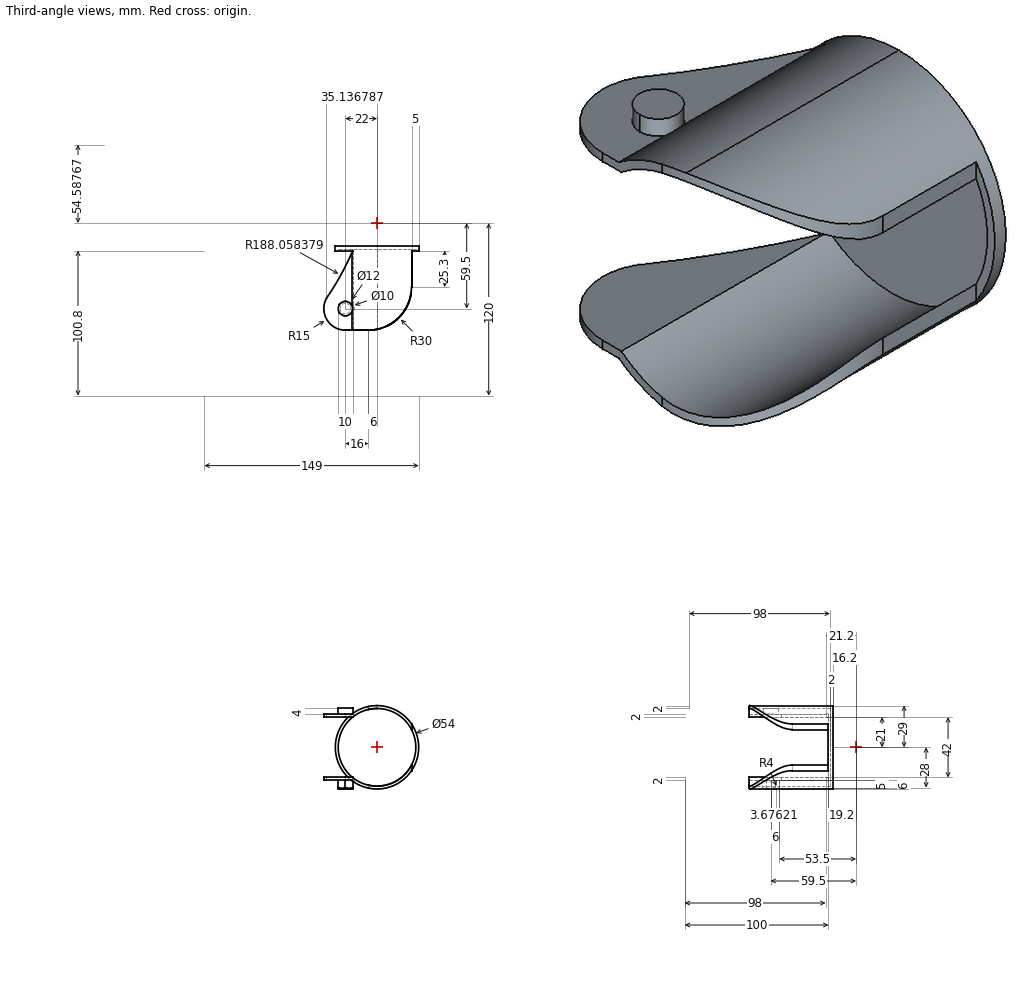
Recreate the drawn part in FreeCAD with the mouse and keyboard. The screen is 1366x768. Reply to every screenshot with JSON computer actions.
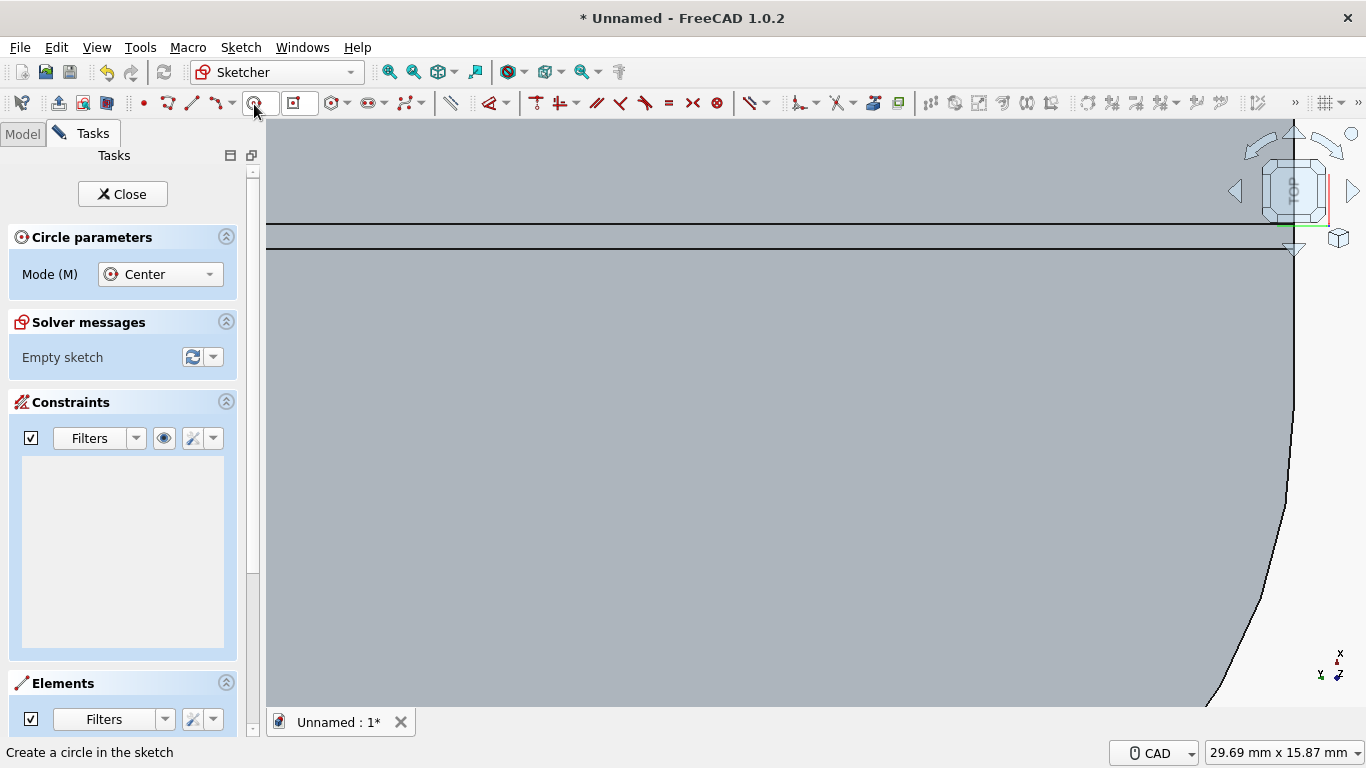
{"action": "left_click", "coordinate": [738, 410]}
{"action": "left_click", "coordinate": [869, 279]}
{"action": "key", "text": "Escape"}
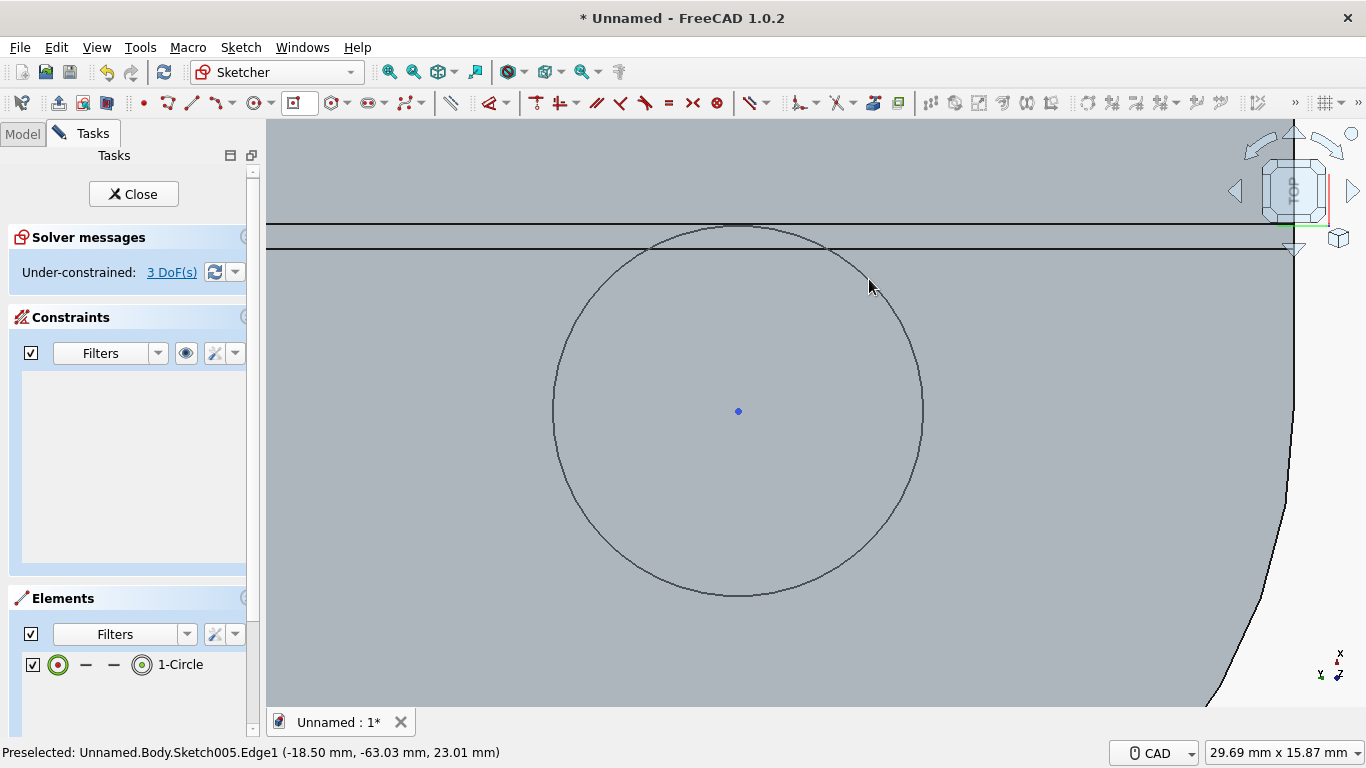
{"action": "left_click", "coordinate": [490, 104]}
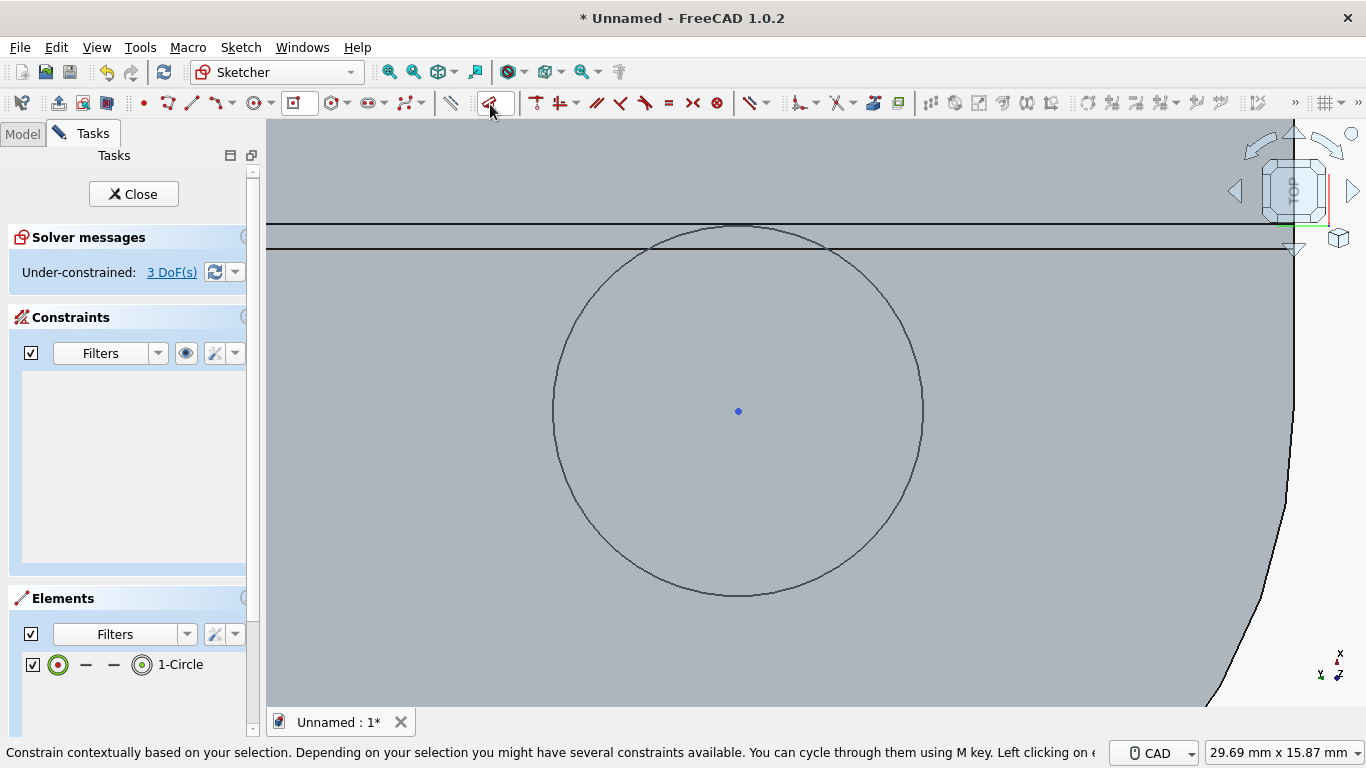
{"action": "left_click", "coordinate": [869, 280]}
{"action": "left_click", "coordinate": [892, 257]}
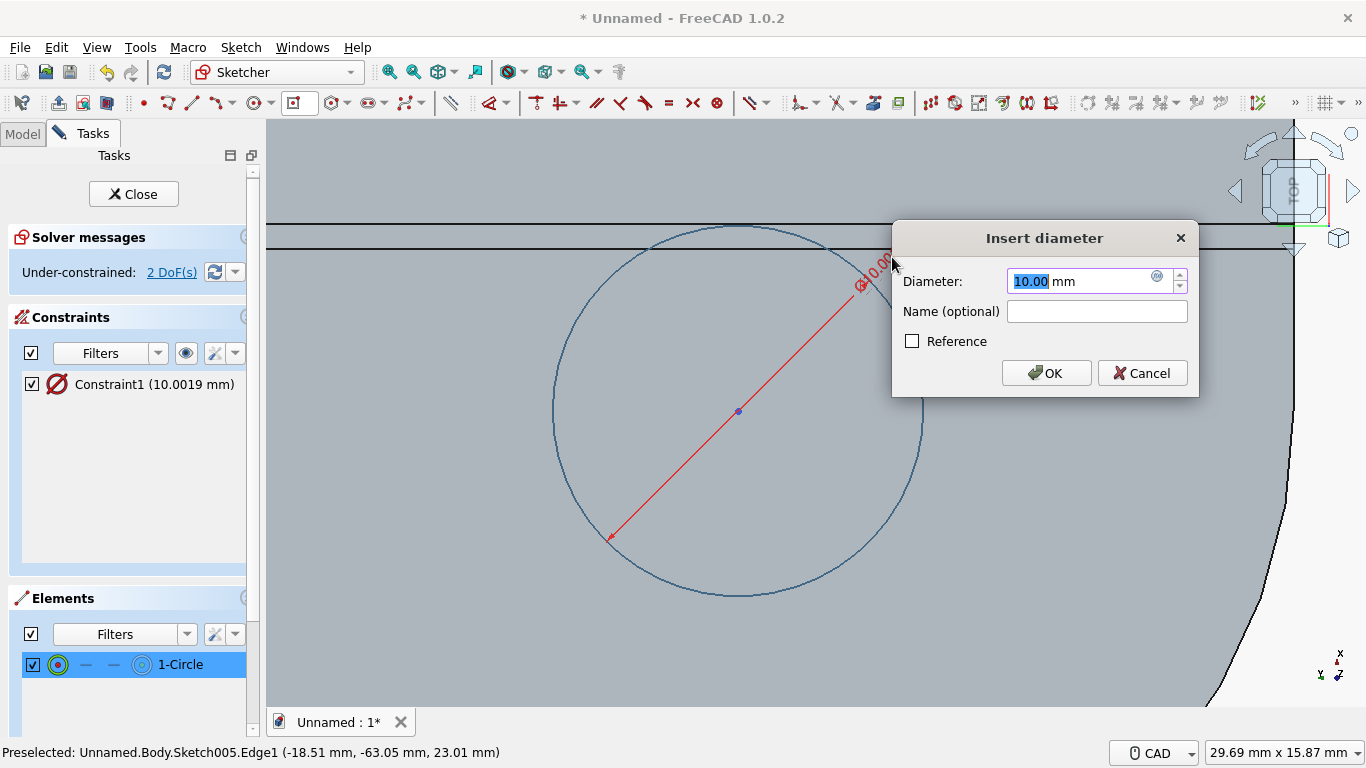
{"action": "type", "text": "10"}
{"action": "key", "text": "Return"}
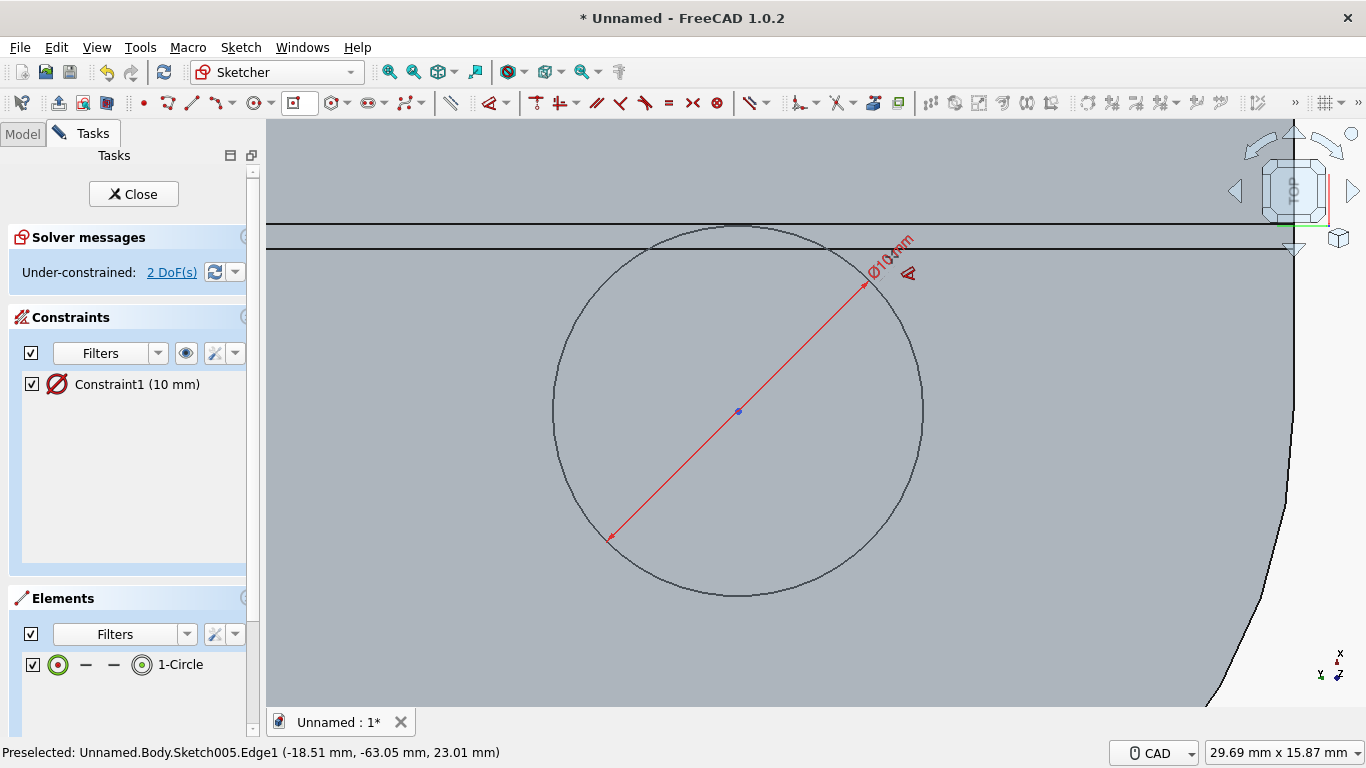
{"action": "left_click", "coordinate": [738, 411]}
{"action": "left_click", "coordinate": [772, 279]}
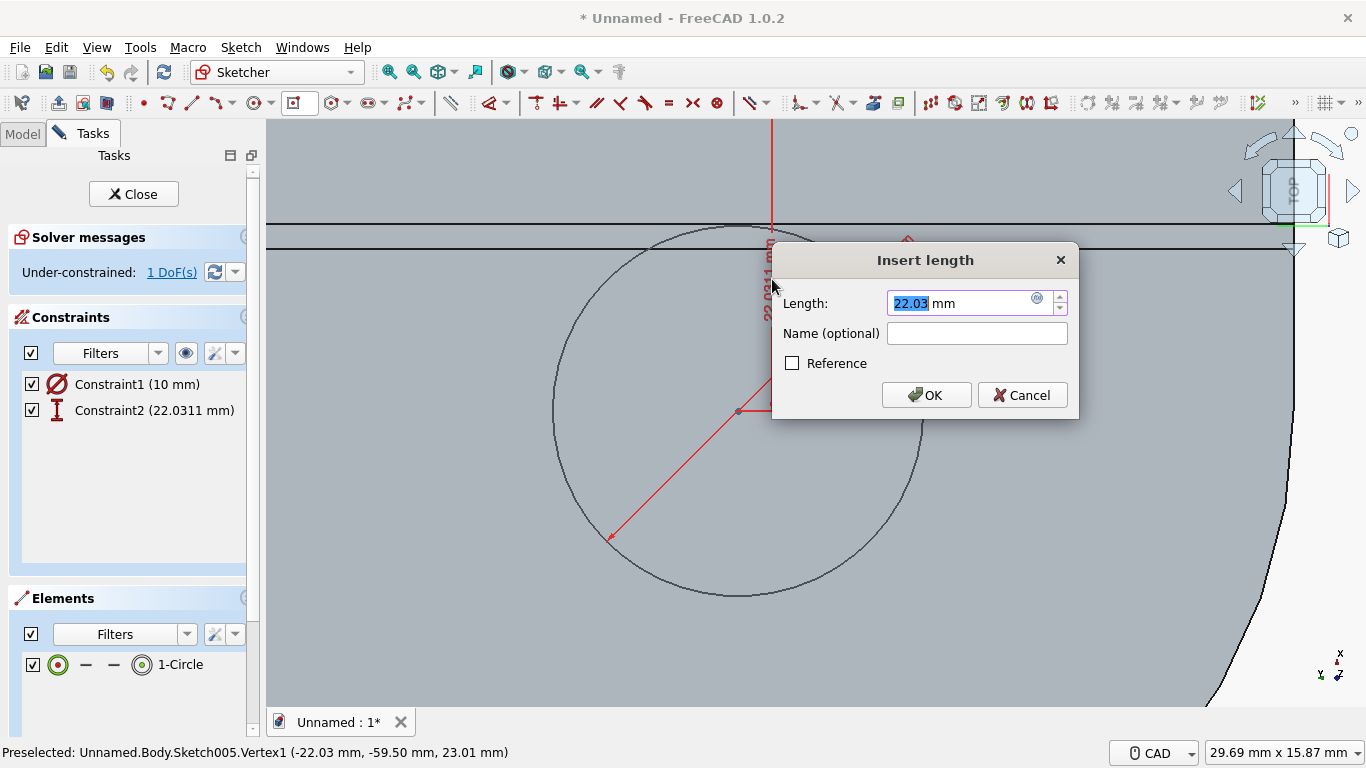
{"action": "type", "text": "22"}
{"action": "key", "text": "Return"}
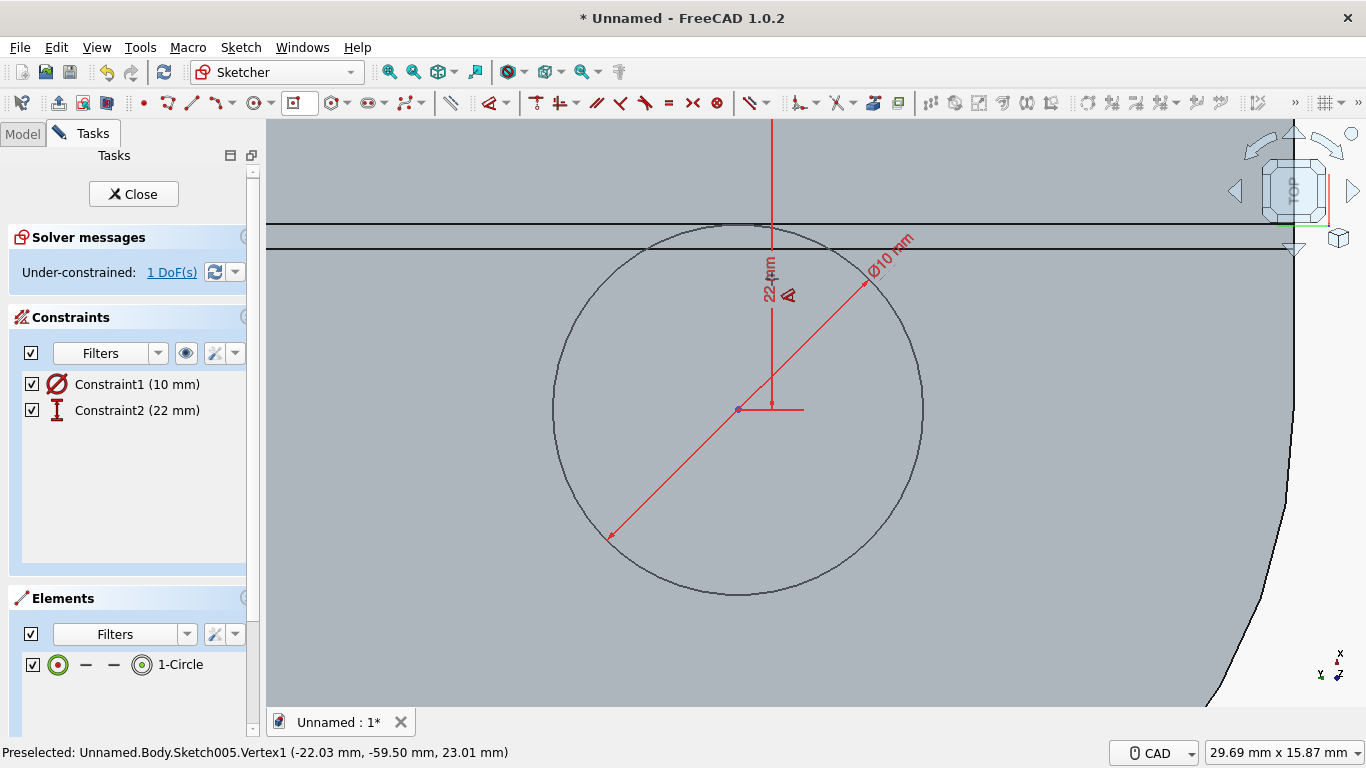
{"action": "left_click", "coordinate": [738, 410]}
{"action": "left_click", "coordinate": [516, 444]}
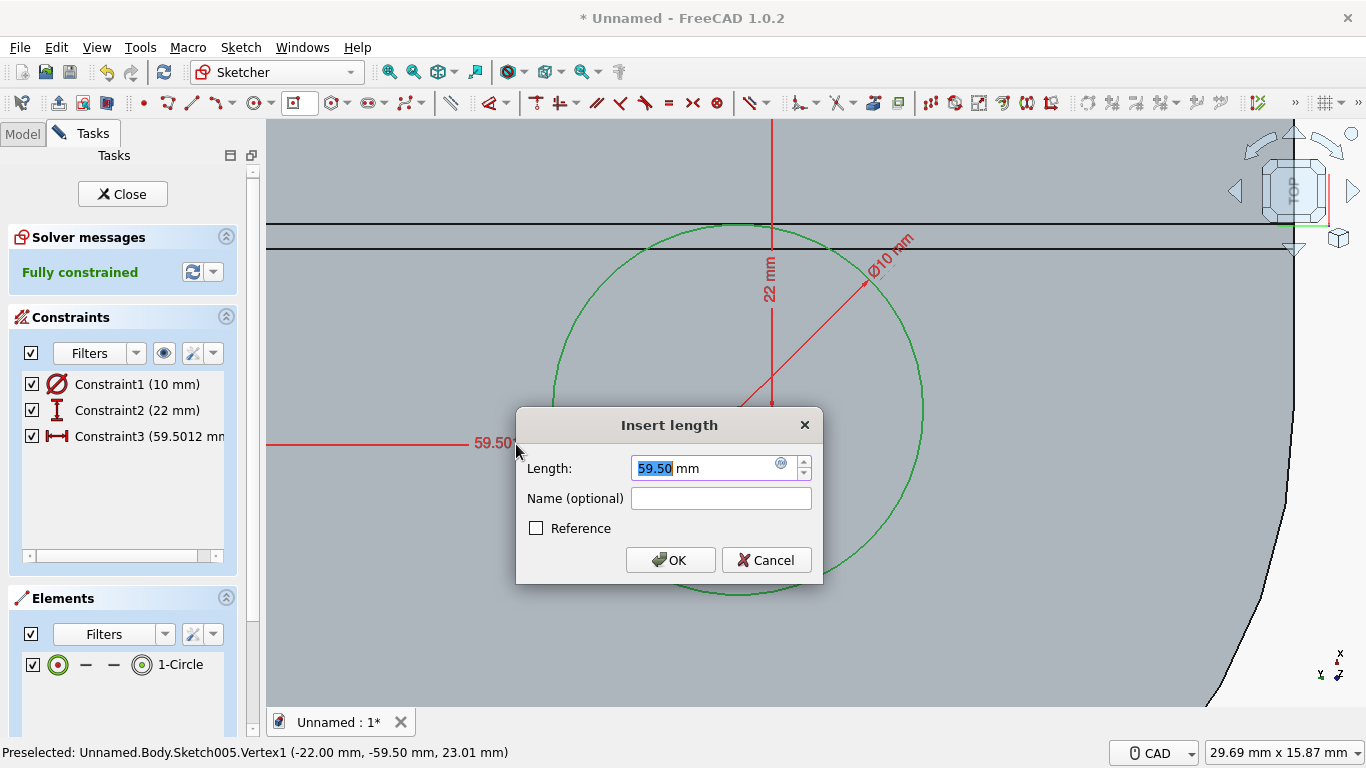
{"action": "type", "text": "59.5"}
{"action": "key", "text": "Return"}
{"action": "key", "text": "Escape"}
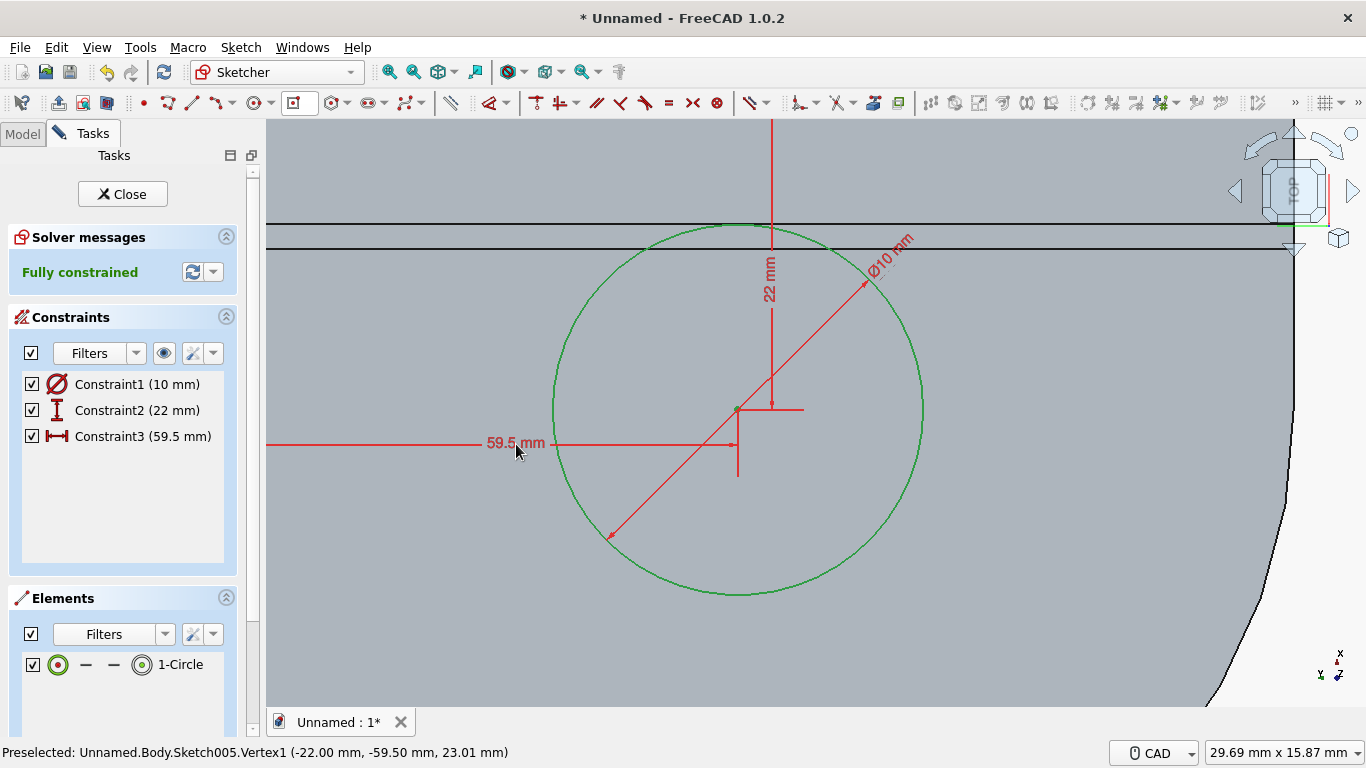
{"action": "left_click", "coordinate": [123, 194]}